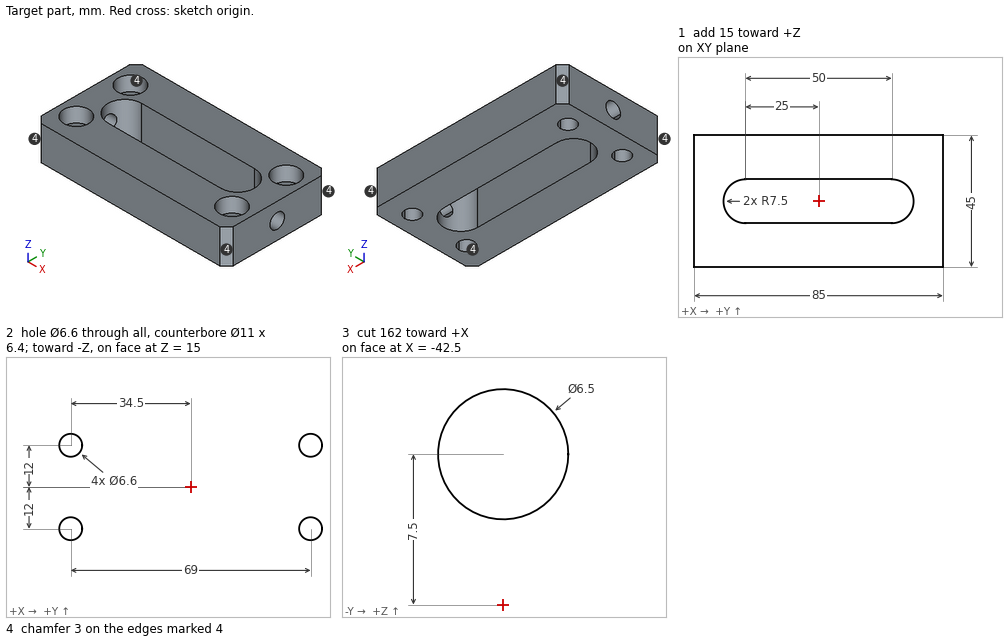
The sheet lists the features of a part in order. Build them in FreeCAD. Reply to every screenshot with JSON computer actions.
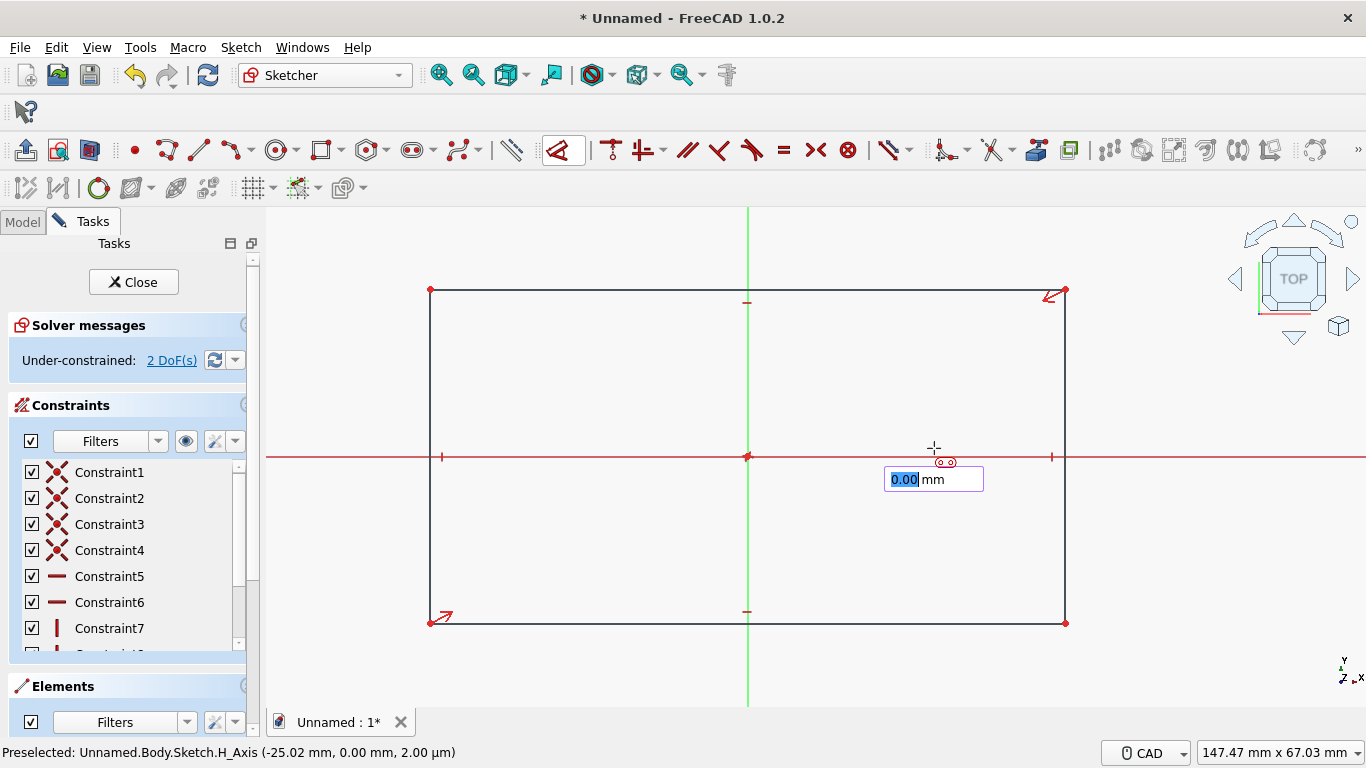
{"action": "left_click", "coordinate": [692, 401]}
{"action": "key", "text": "Escape"}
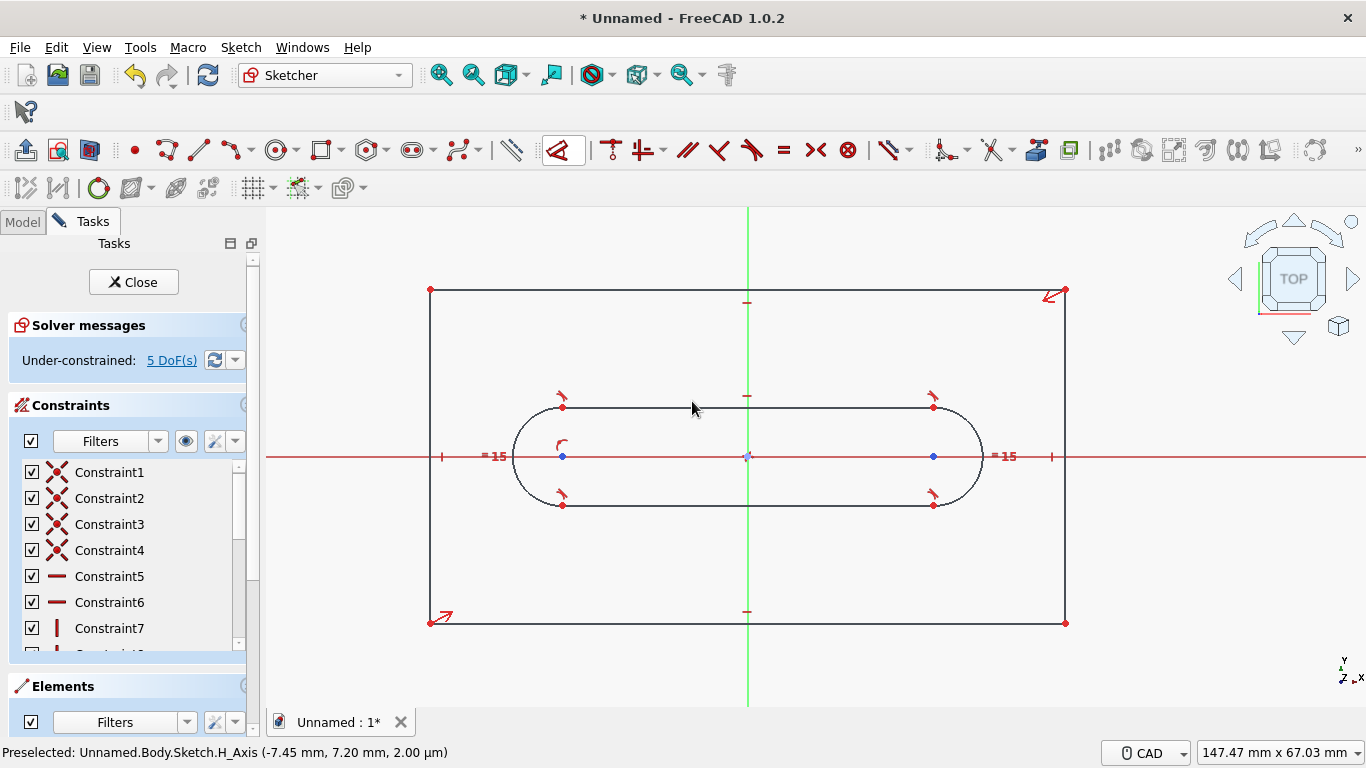
{"action": "key", "text": "d"}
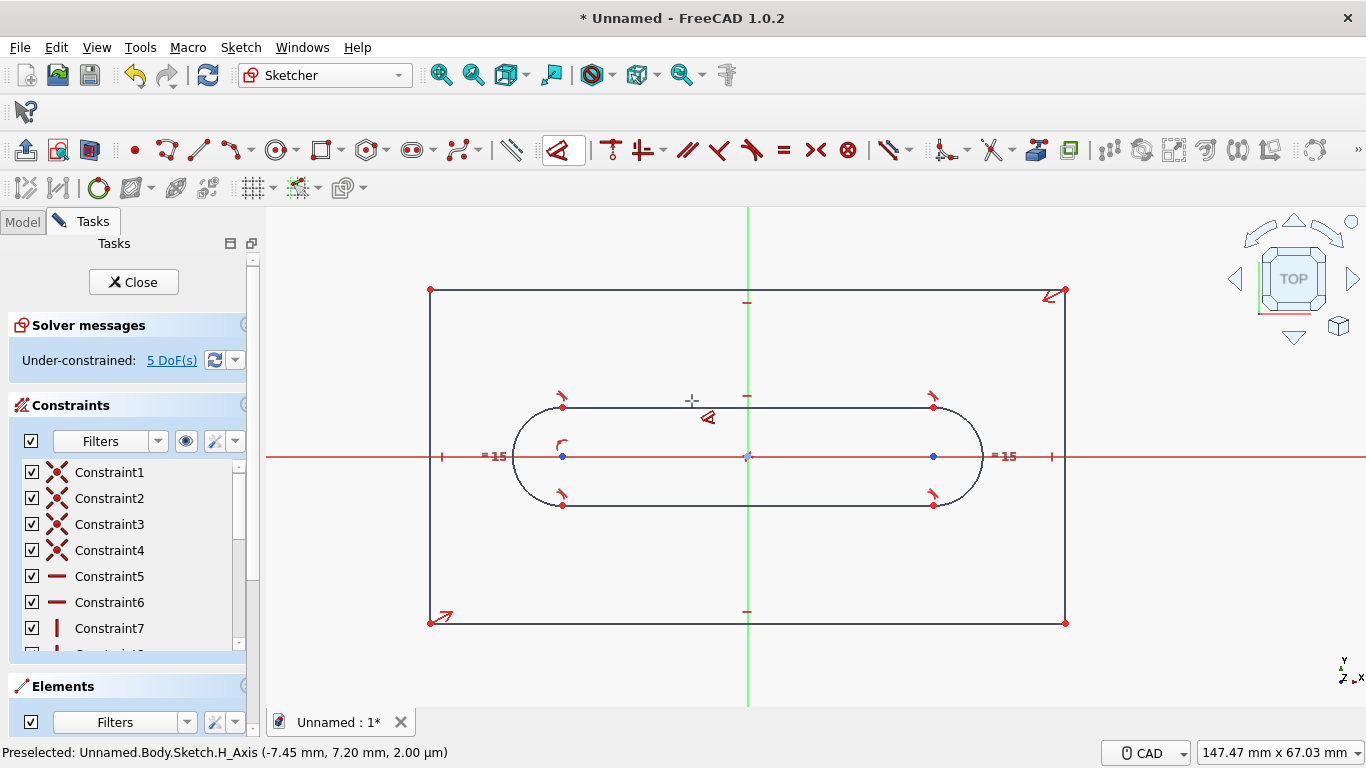
{"action": "left_click", "coordinate": [522, 428]}
{"action": "left_click", "coordinate": [496, 409]}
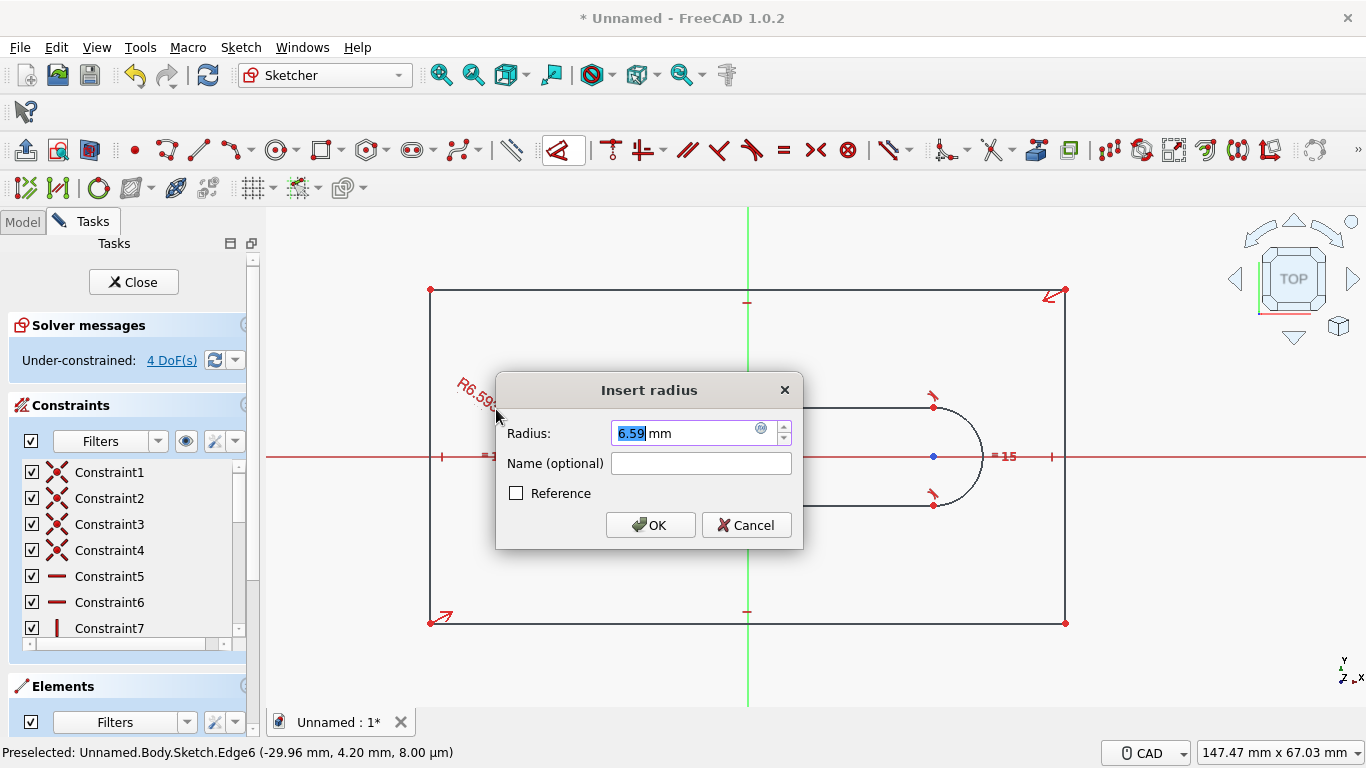
{"action": "type", "text": "7.5"}
{"action": "key", "text": "Return"}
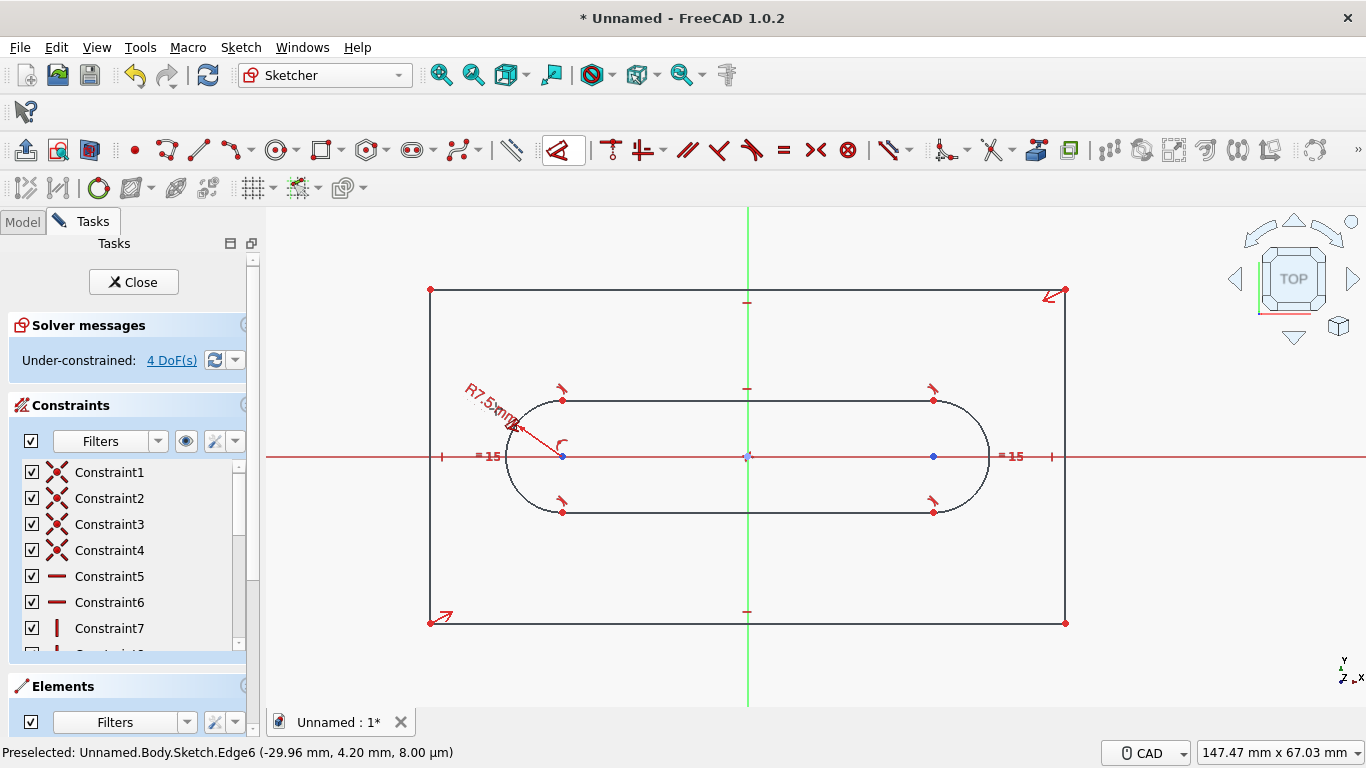
{"action": "left_click", "coordinate": [621, 624]}
{"action": "left_click", "coordinate": [602, 658]}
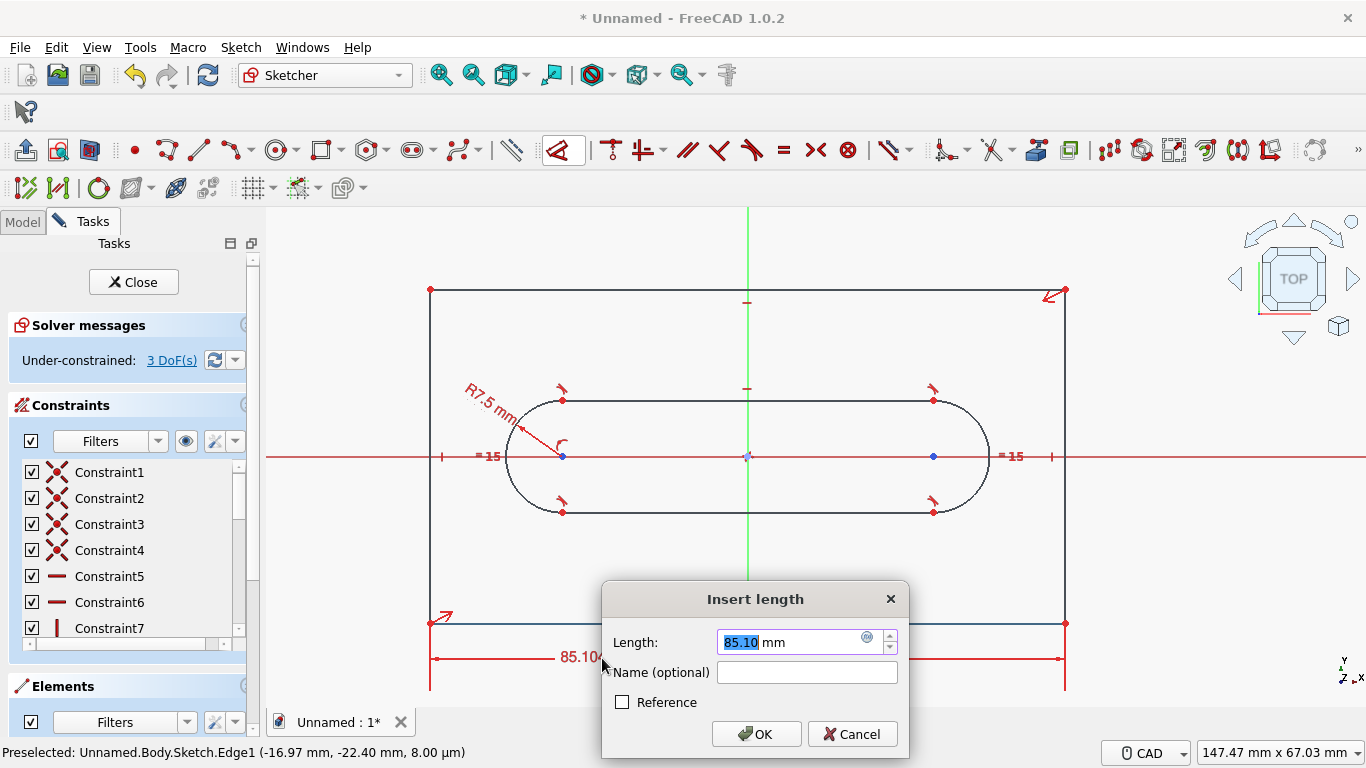
{"action": "type", "text": "85"}
{"action": "key", "text": "Return"}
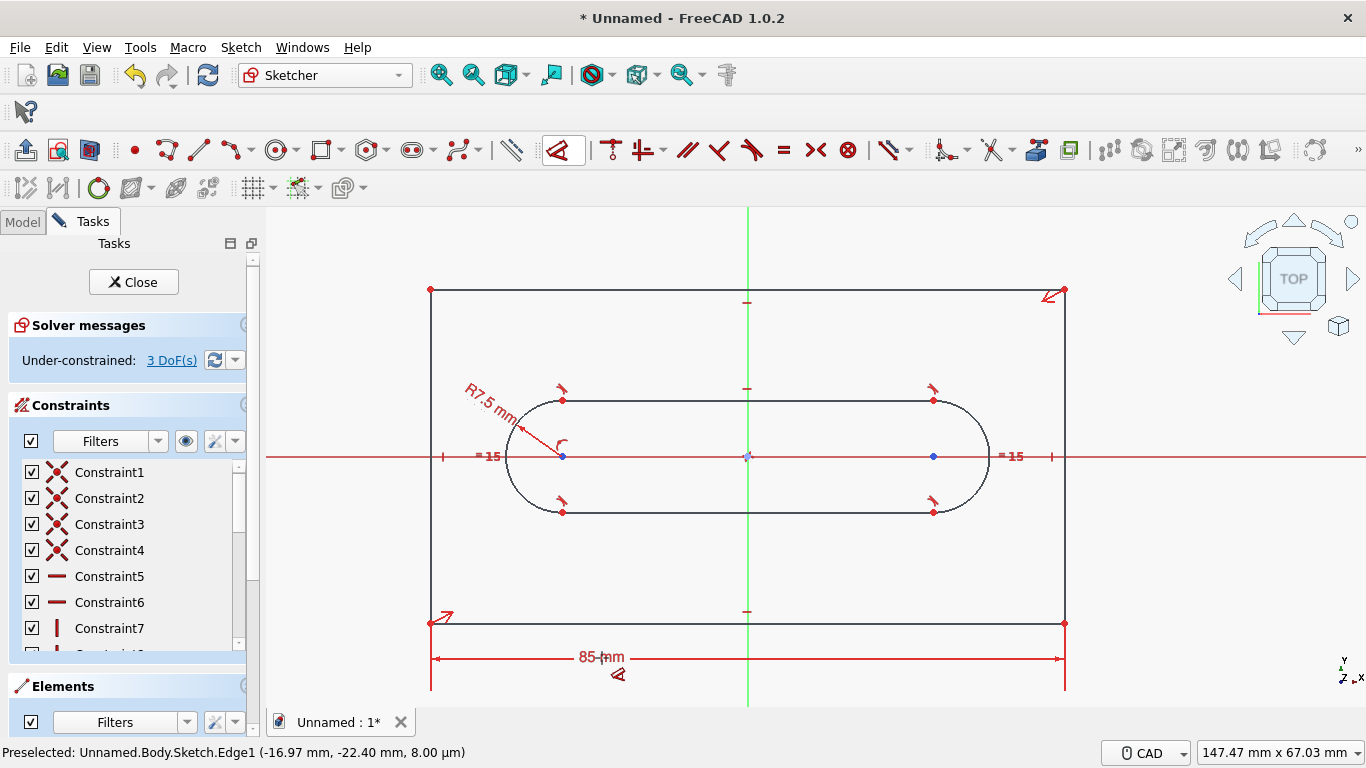
{"action": "left_click", "coordinate": [1065, 524]}
{"action": "left_click", "coordinate": [1099, 380]}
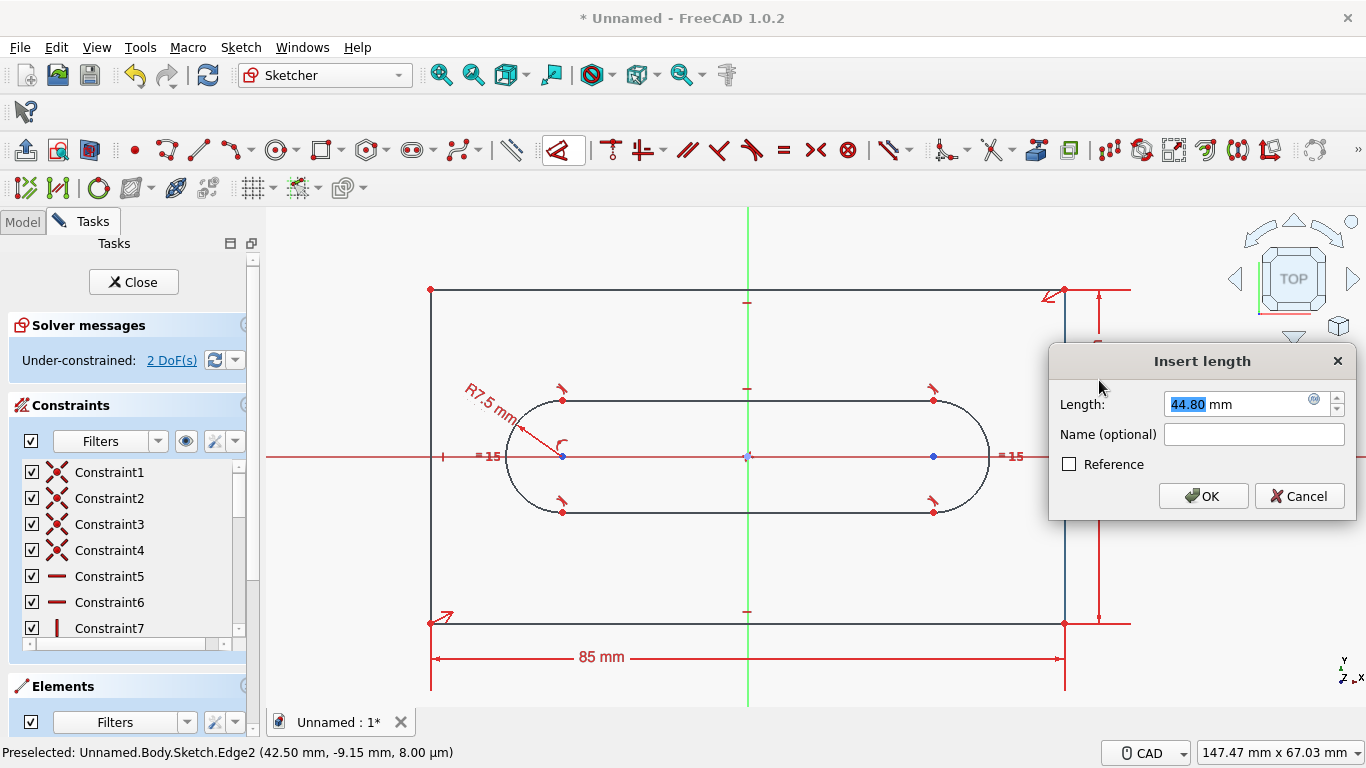
{"action": "type", "text": "45"}
{"action": "key", "text": "Return"}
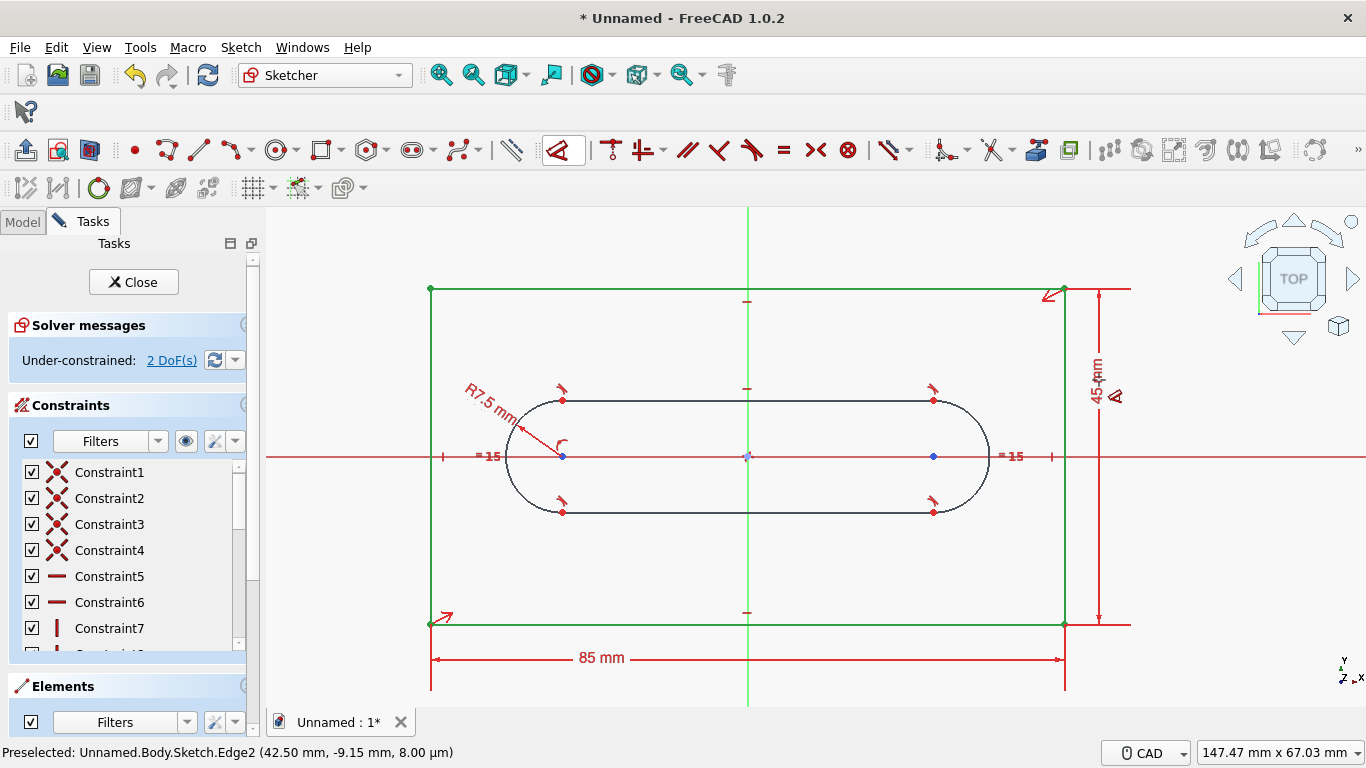
{"action": "left_click", "coordinate": [673, 401]}
{"action": "left_click", "coordinate": [662, 367]}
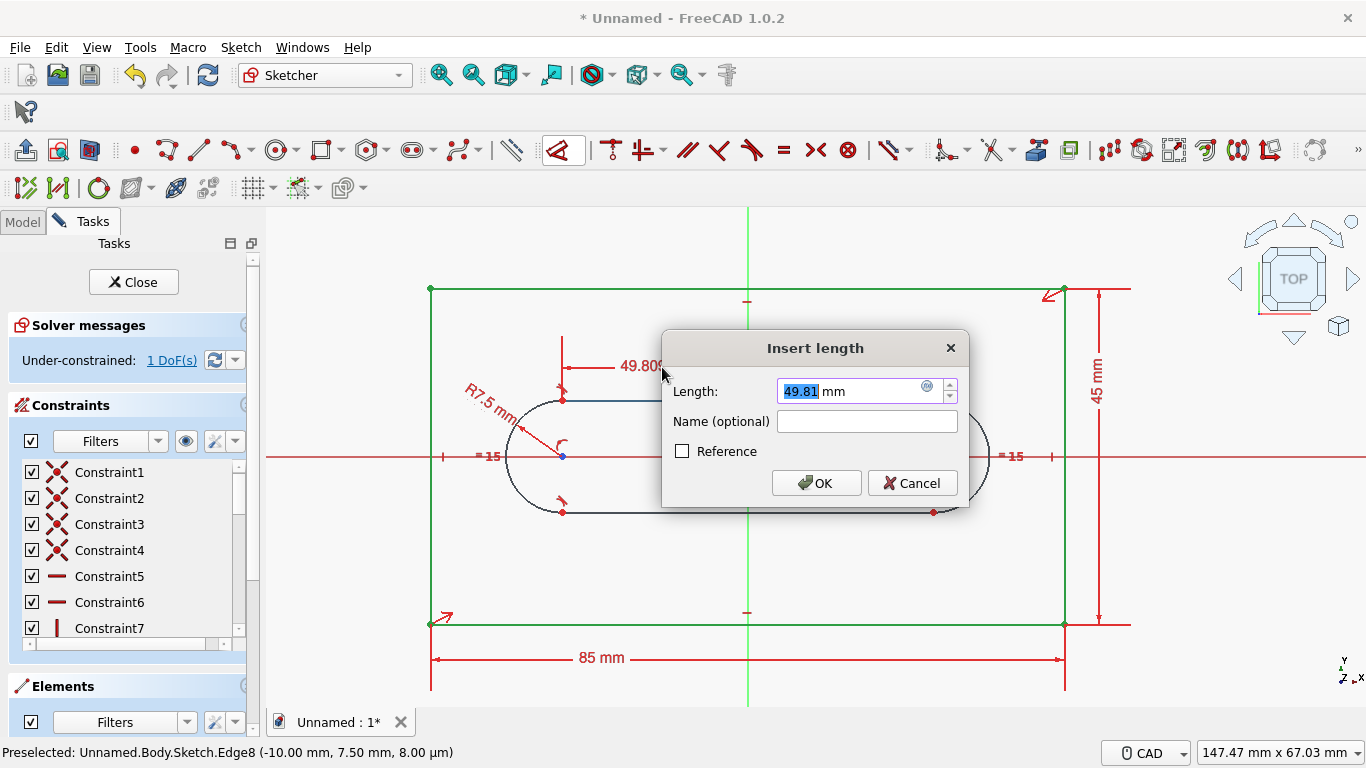
{"action": "type", "text": "50"}
{"action": "key", "text": "Return"}